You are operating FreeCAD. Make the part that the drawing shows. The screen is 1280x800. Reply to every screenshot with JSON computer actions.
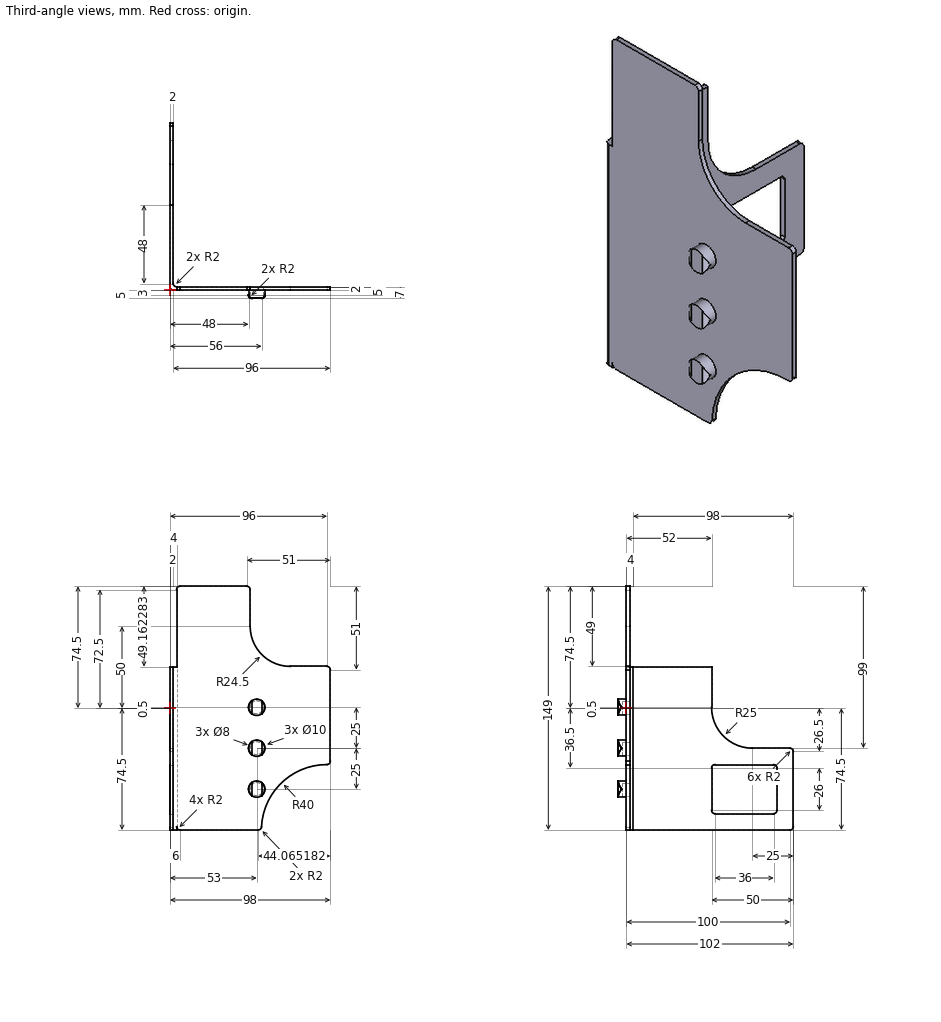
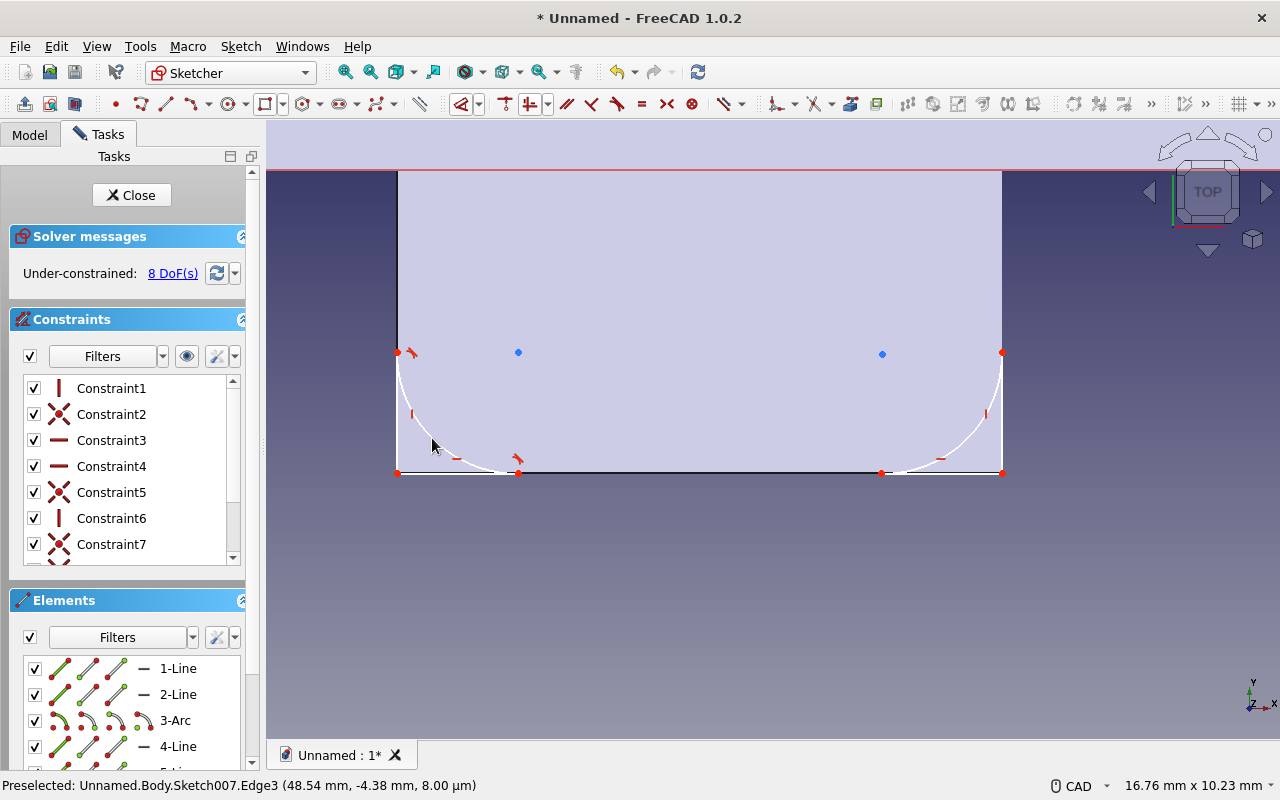
{"action": "left_click", "coordinate": [966, 474]}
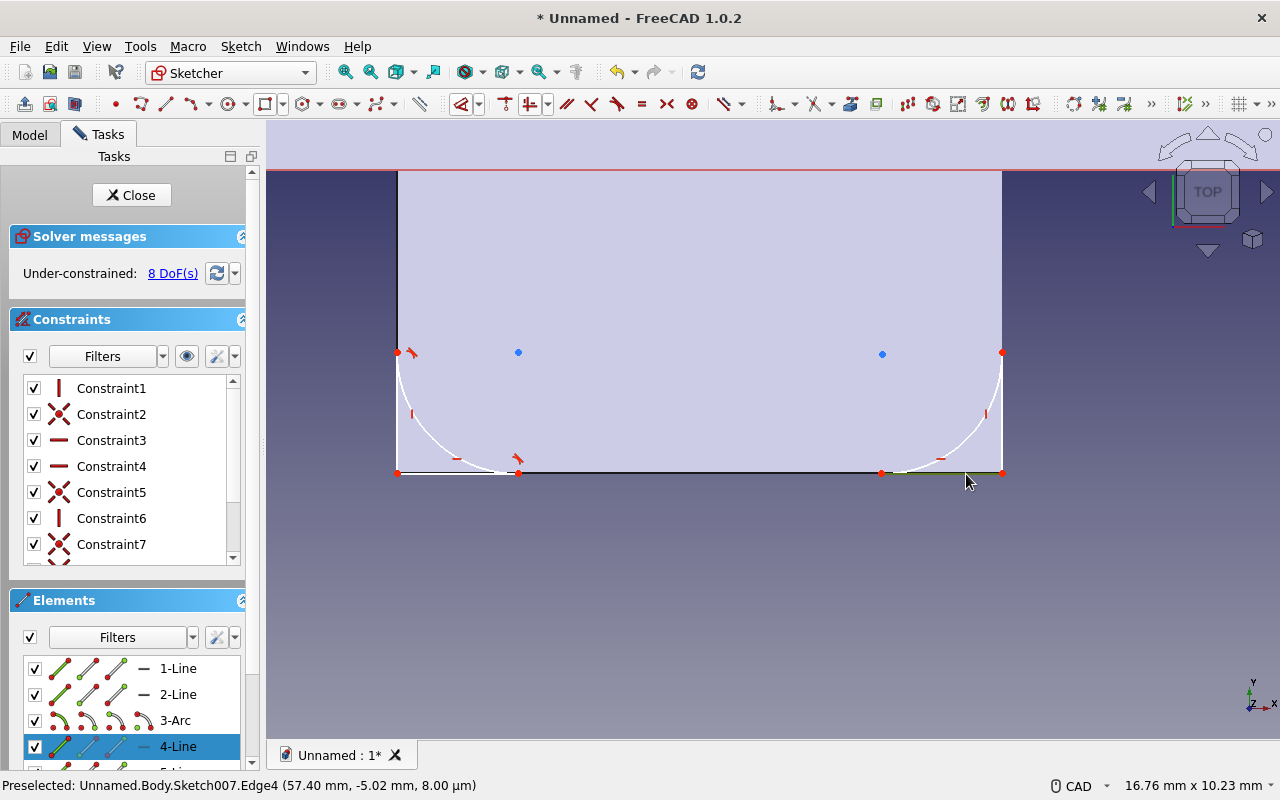
{"action": "left_click", "coordinate": [967, 439]}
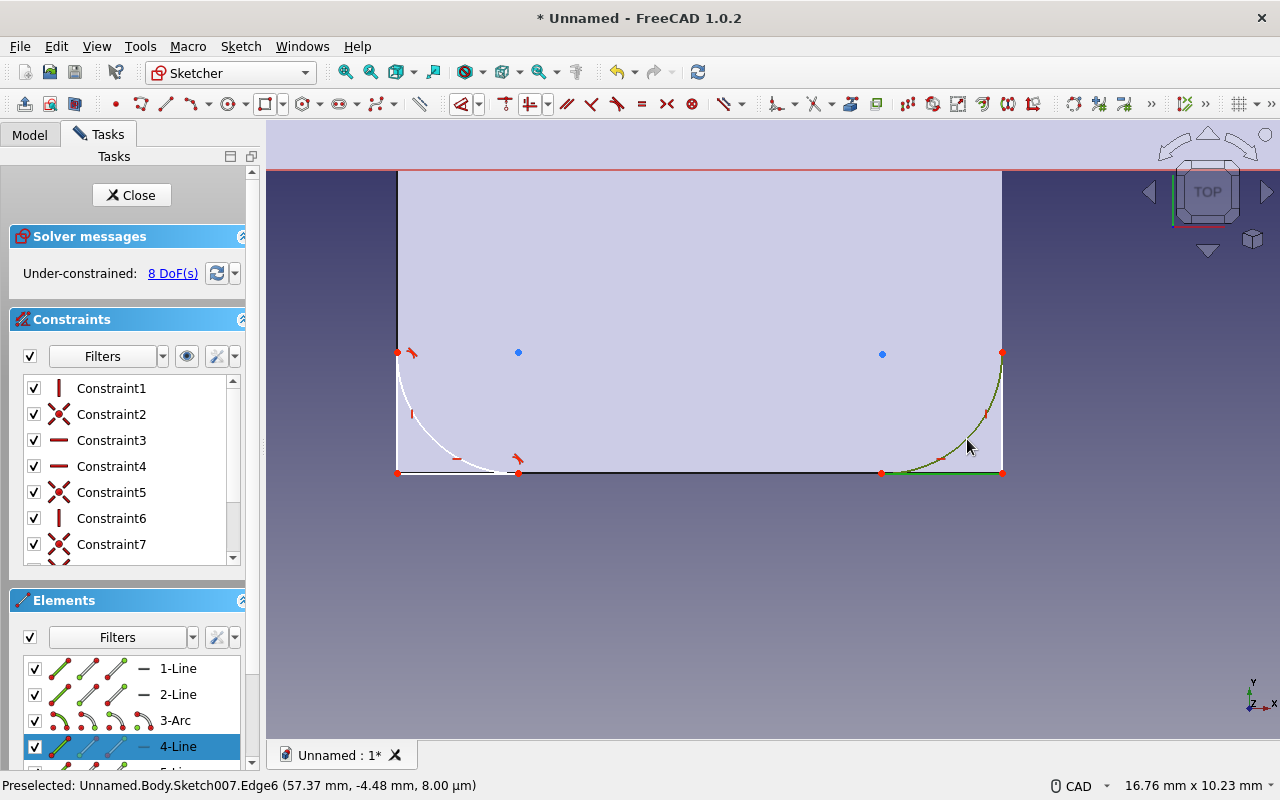
{"action": "key", "text": "t"}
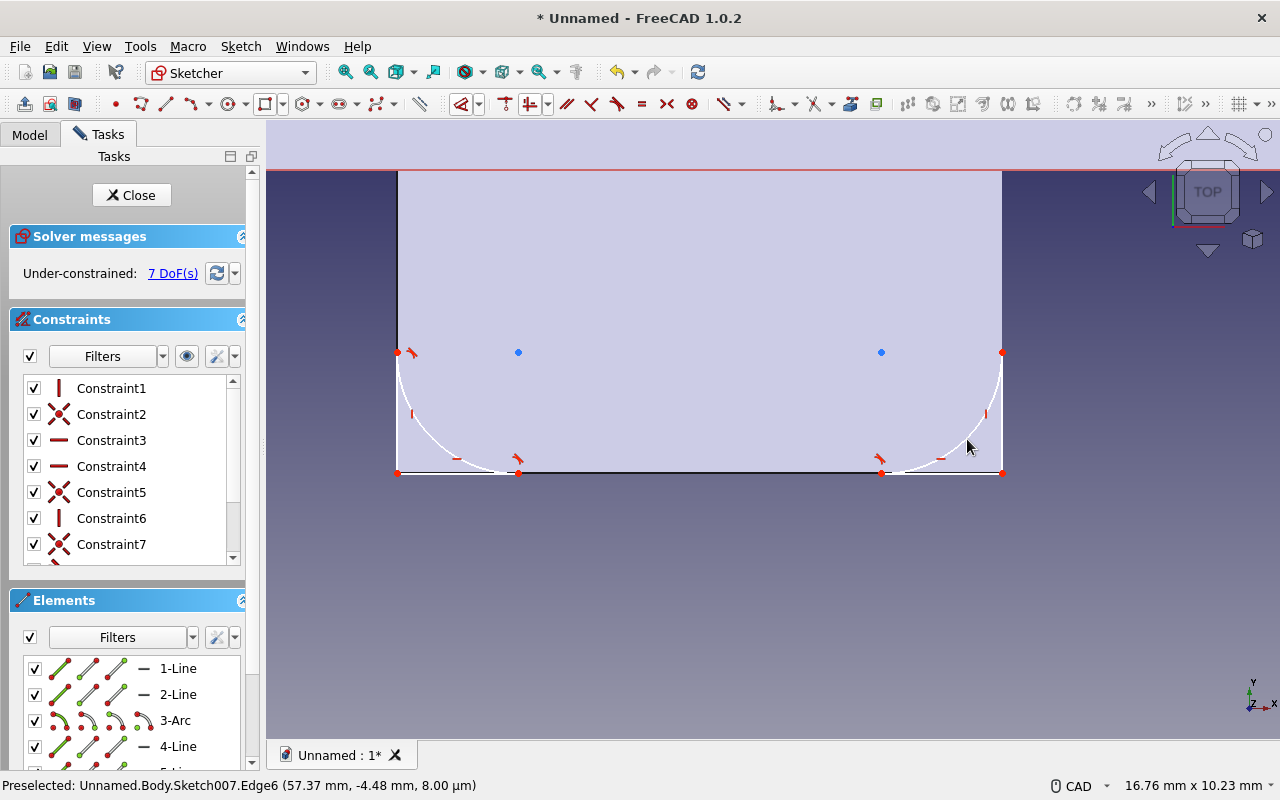
{"action": "left_click", "coordinate": [1002, 438]}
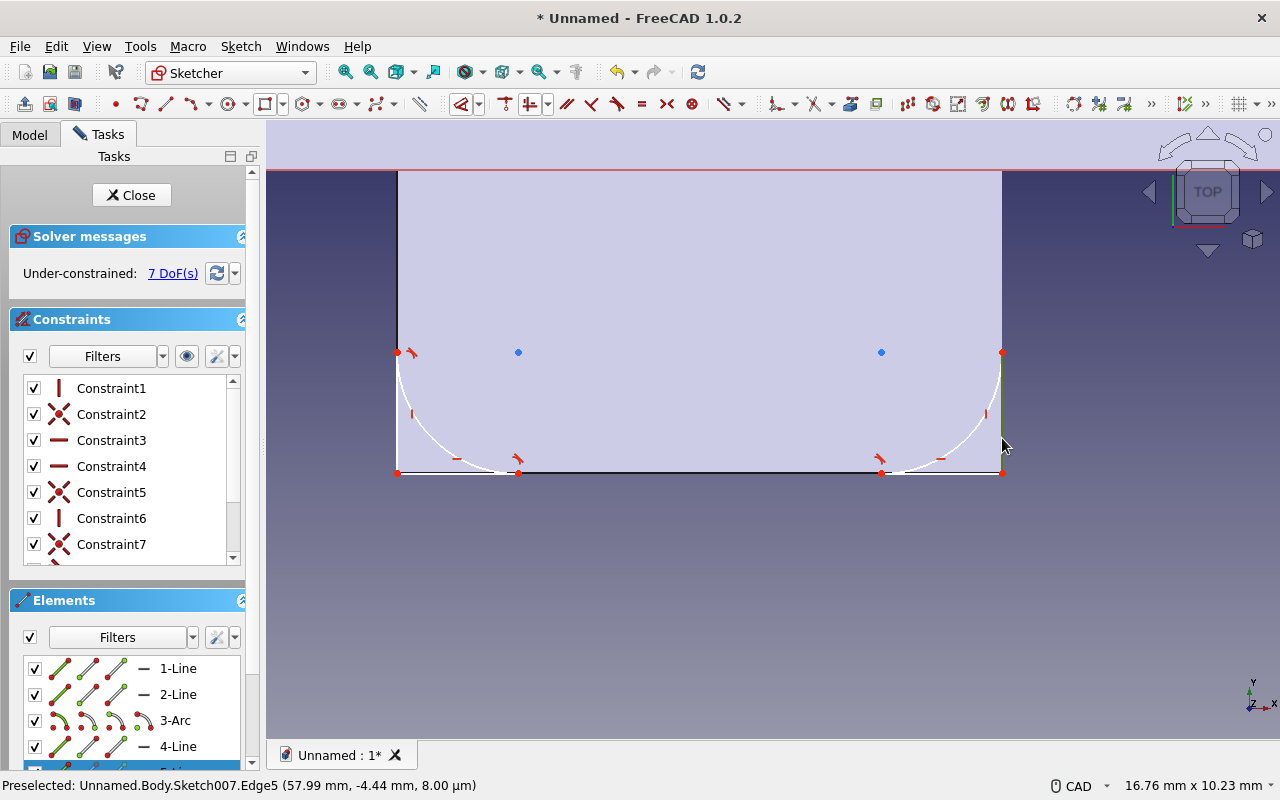
{"action": "left_click", "coordinate": [967, 439]}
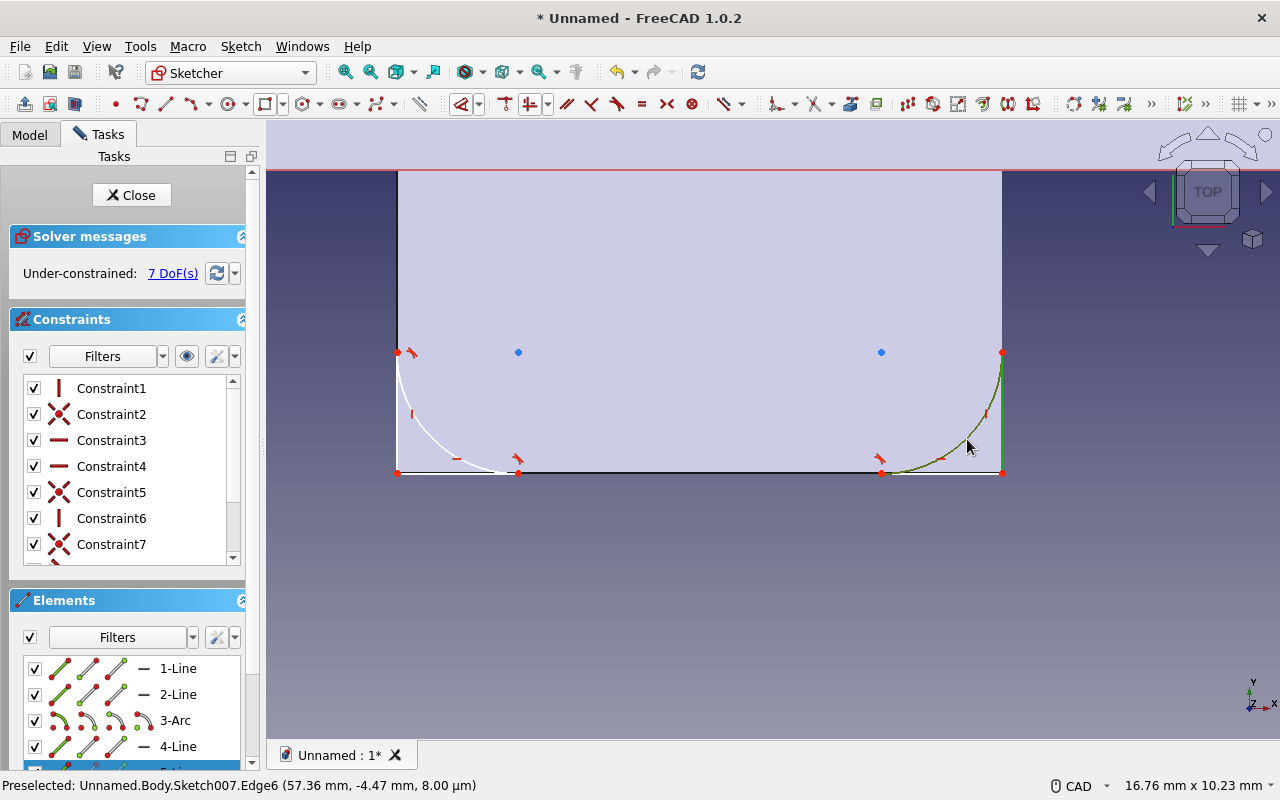
{"action": "key", "text": "t"}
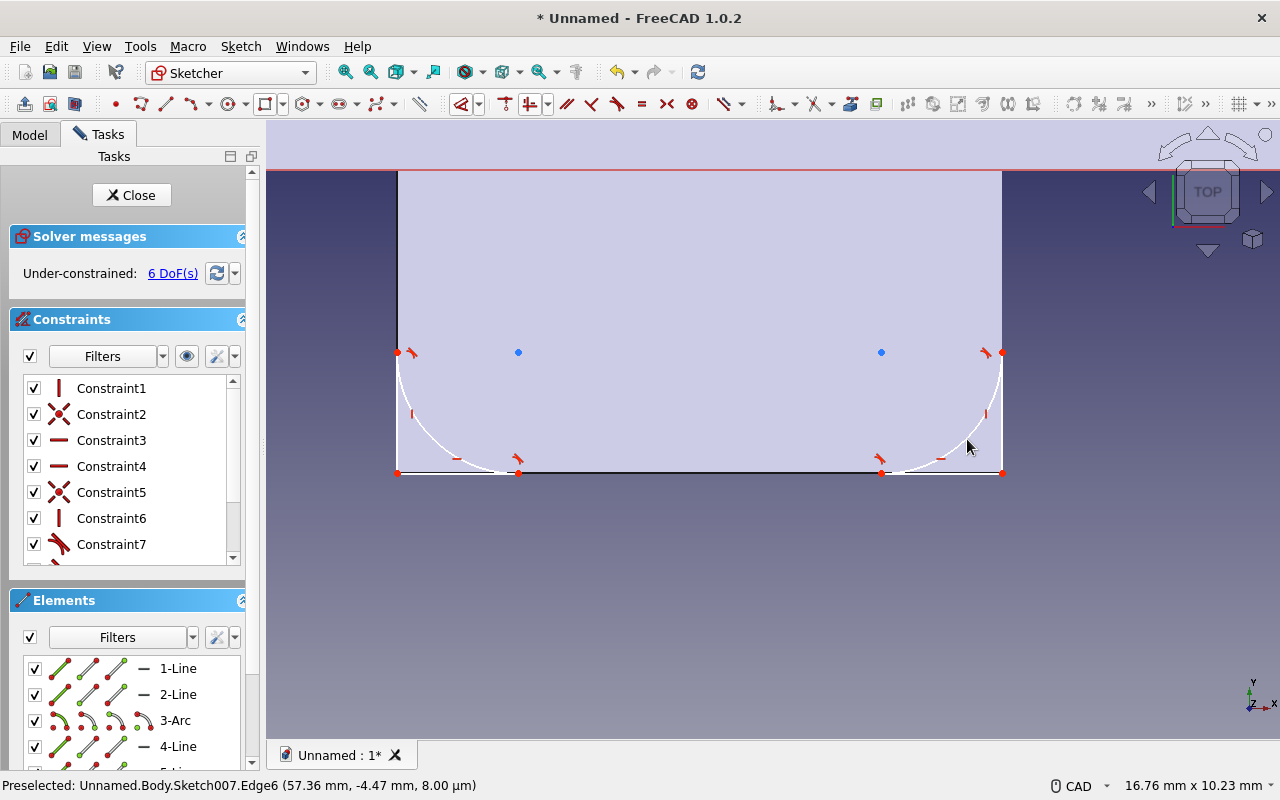
{"action": "left_click", "coordinate": [432, 439]}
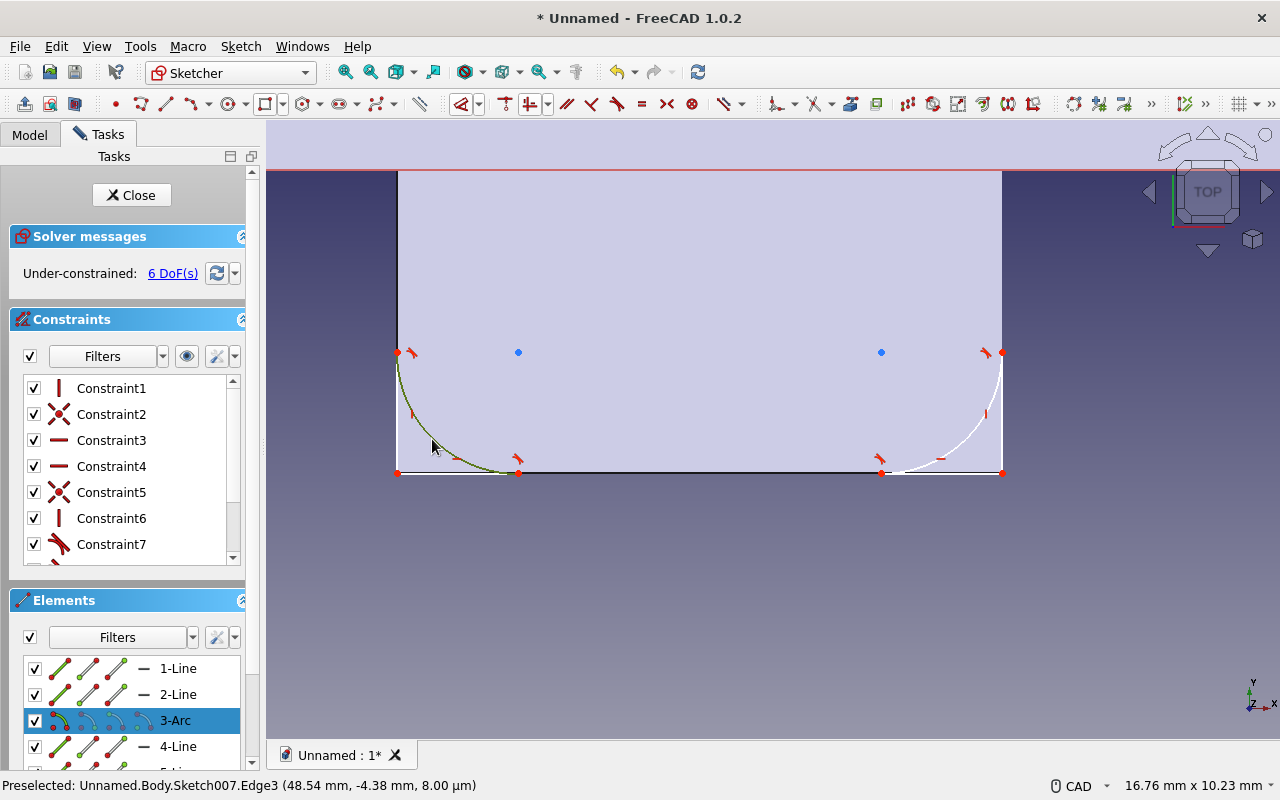
{"action": "left_click", "coordinate": [967, 439]}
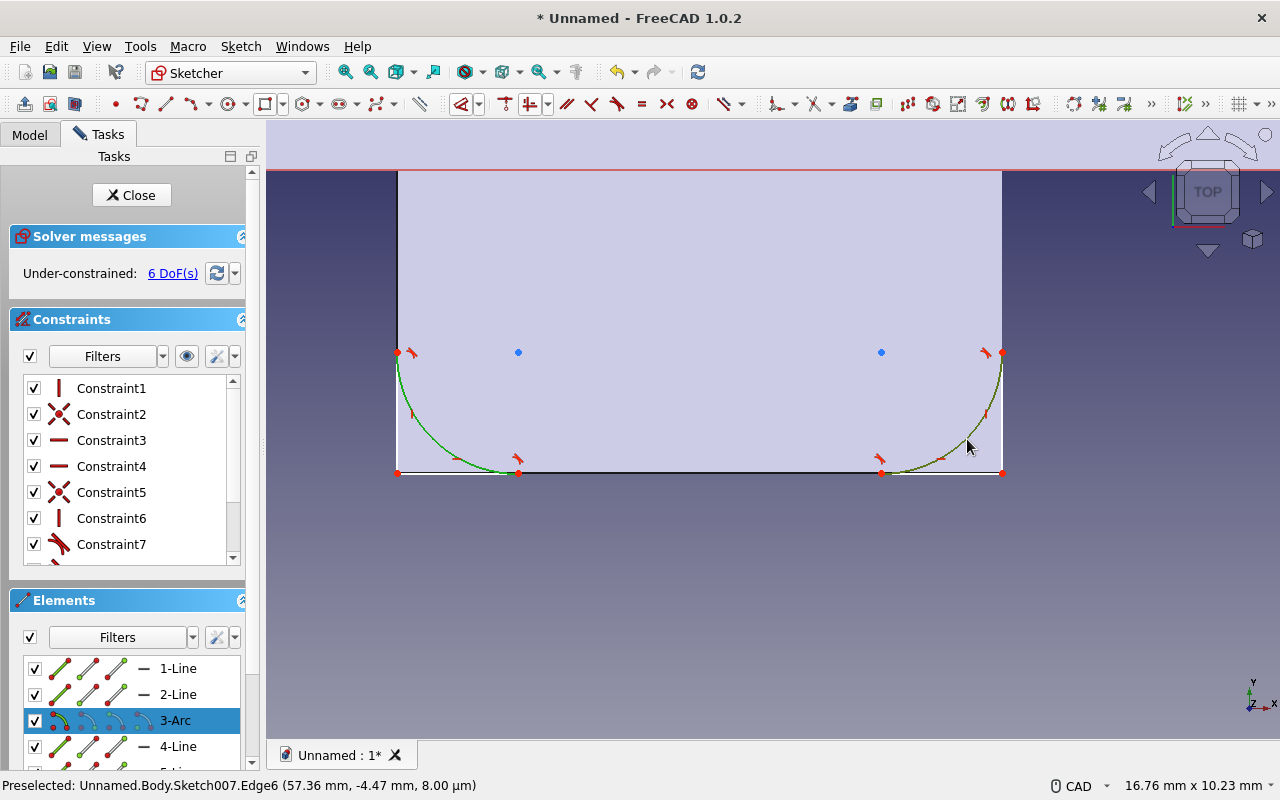
{"action": "key", "text": "e"}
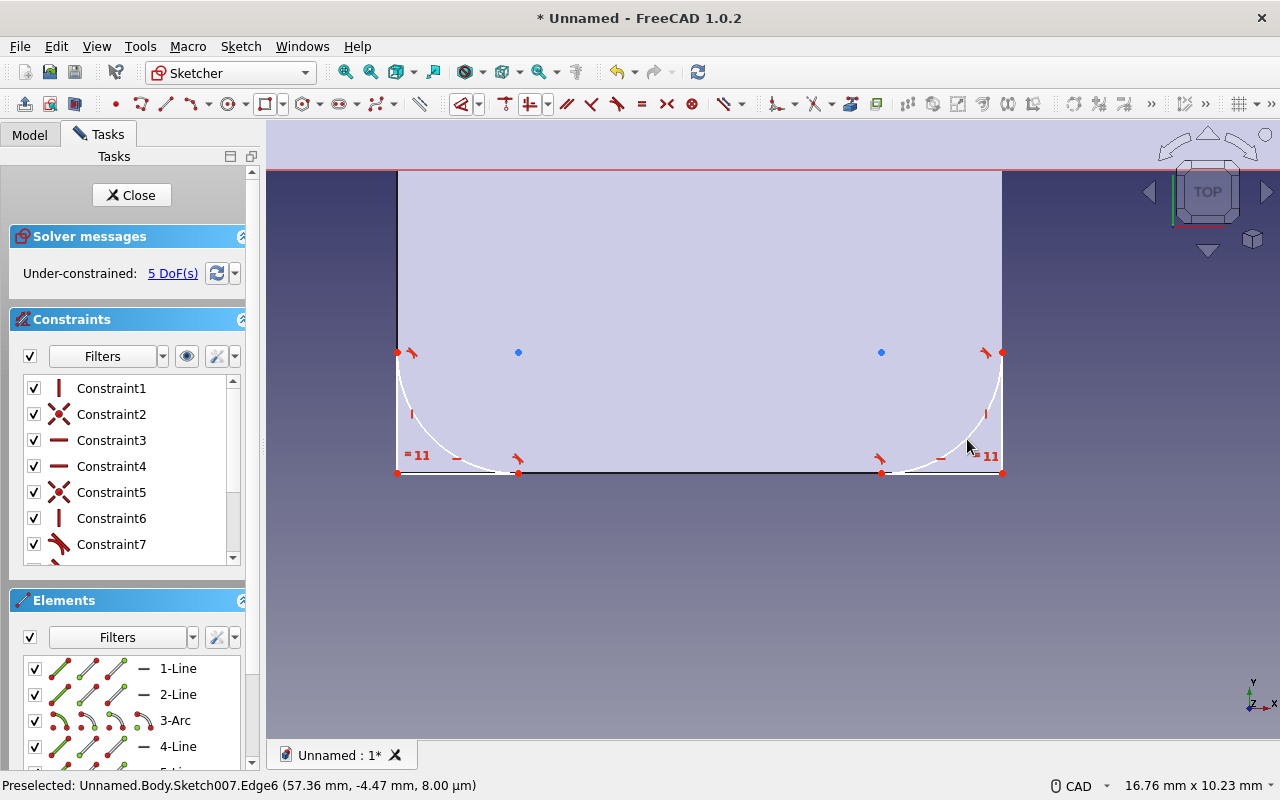
{"action": "left_click", "coordinate": [433, 438]}